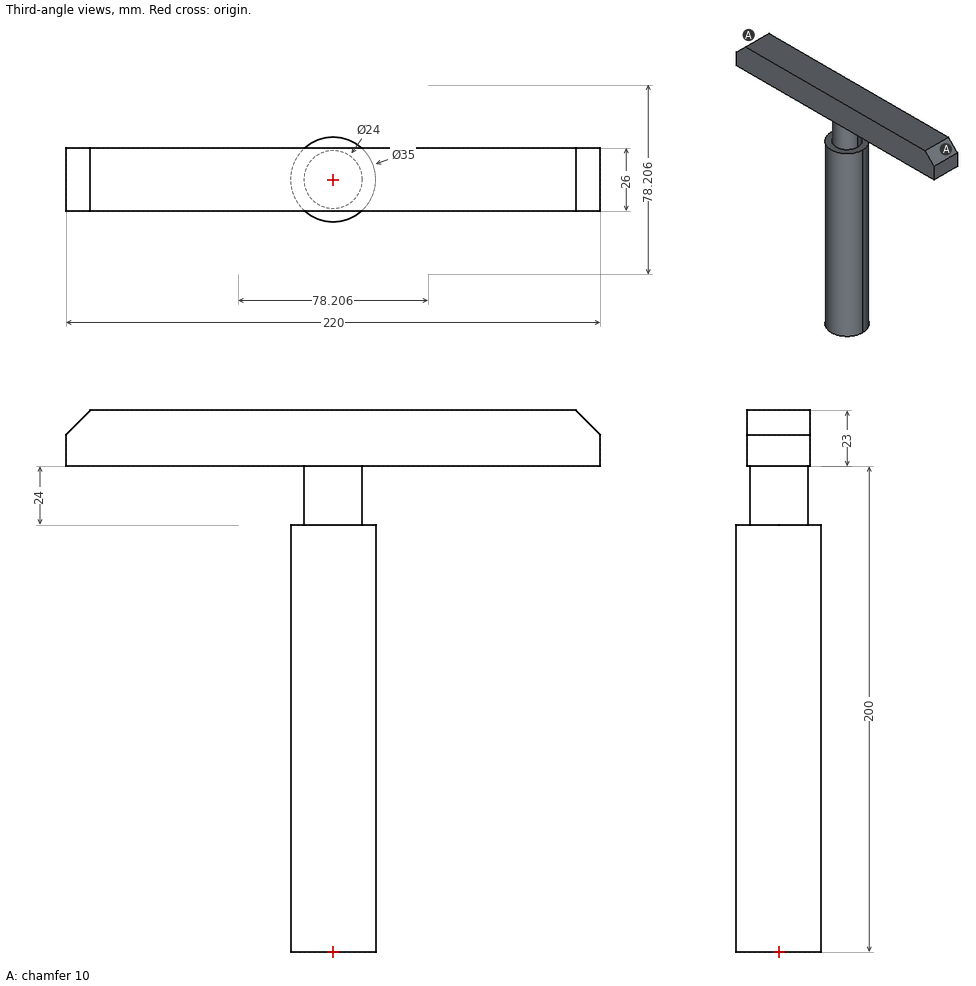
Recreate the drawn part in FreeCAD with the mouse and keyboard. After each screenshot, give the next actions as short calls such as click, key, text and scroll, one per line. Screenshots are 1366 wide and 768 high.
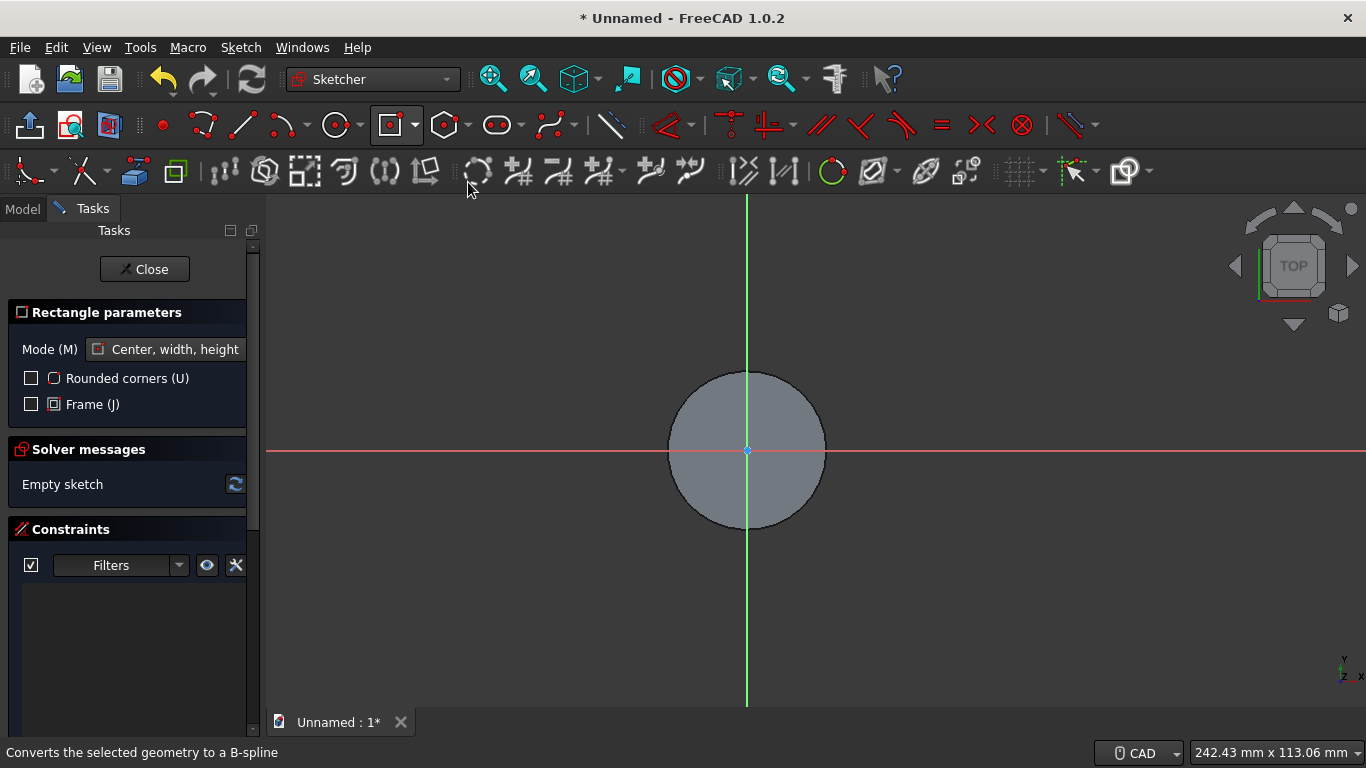
click(747, 450)
click(925, 273)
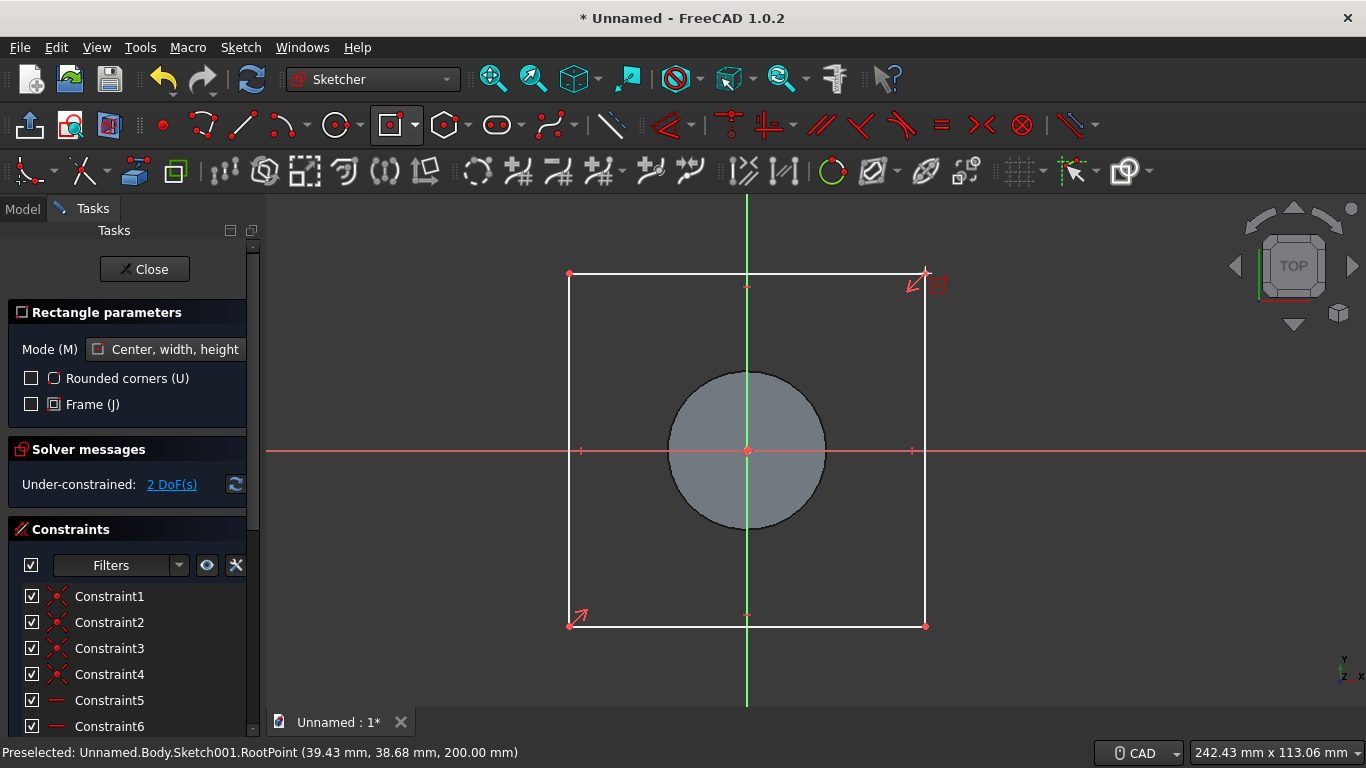
click(336, 126)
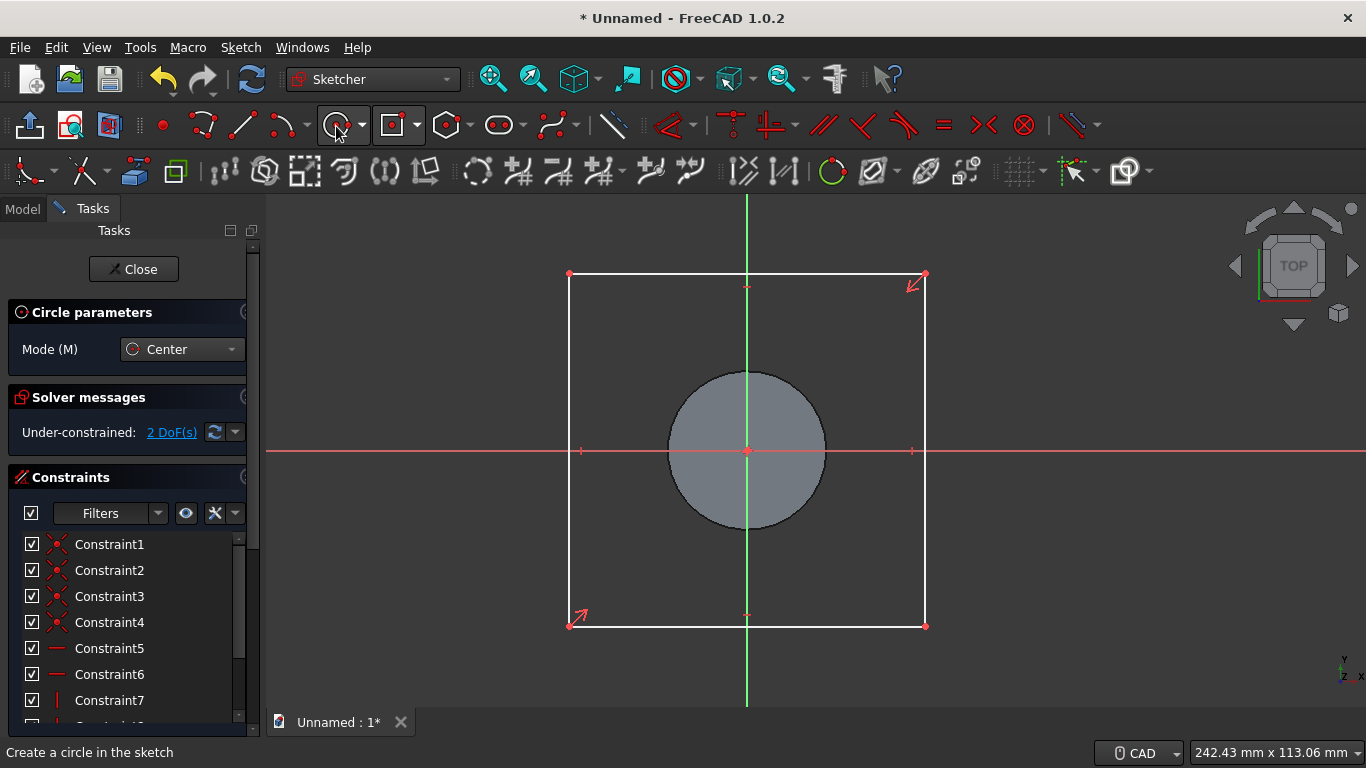
click(747, 450)
click(786, 412)
key(Escape)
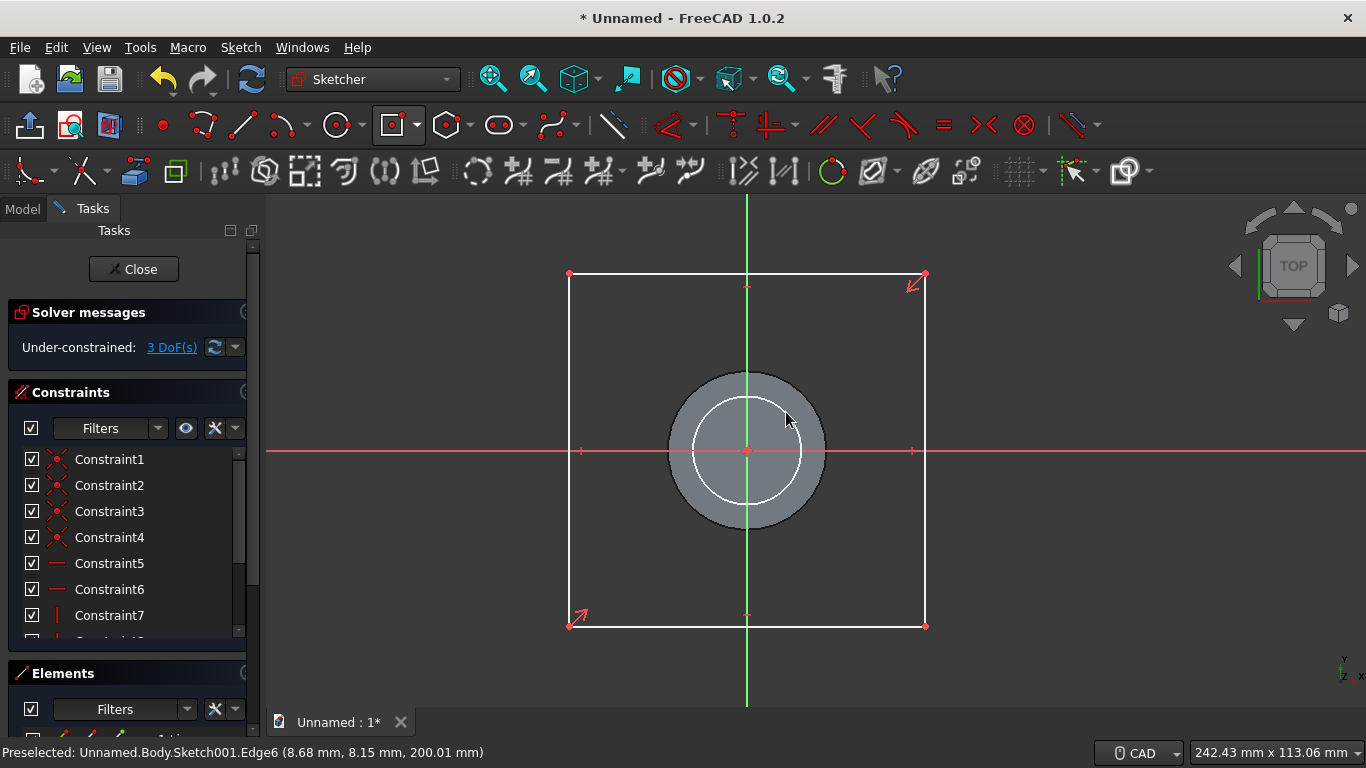
click(668, 126)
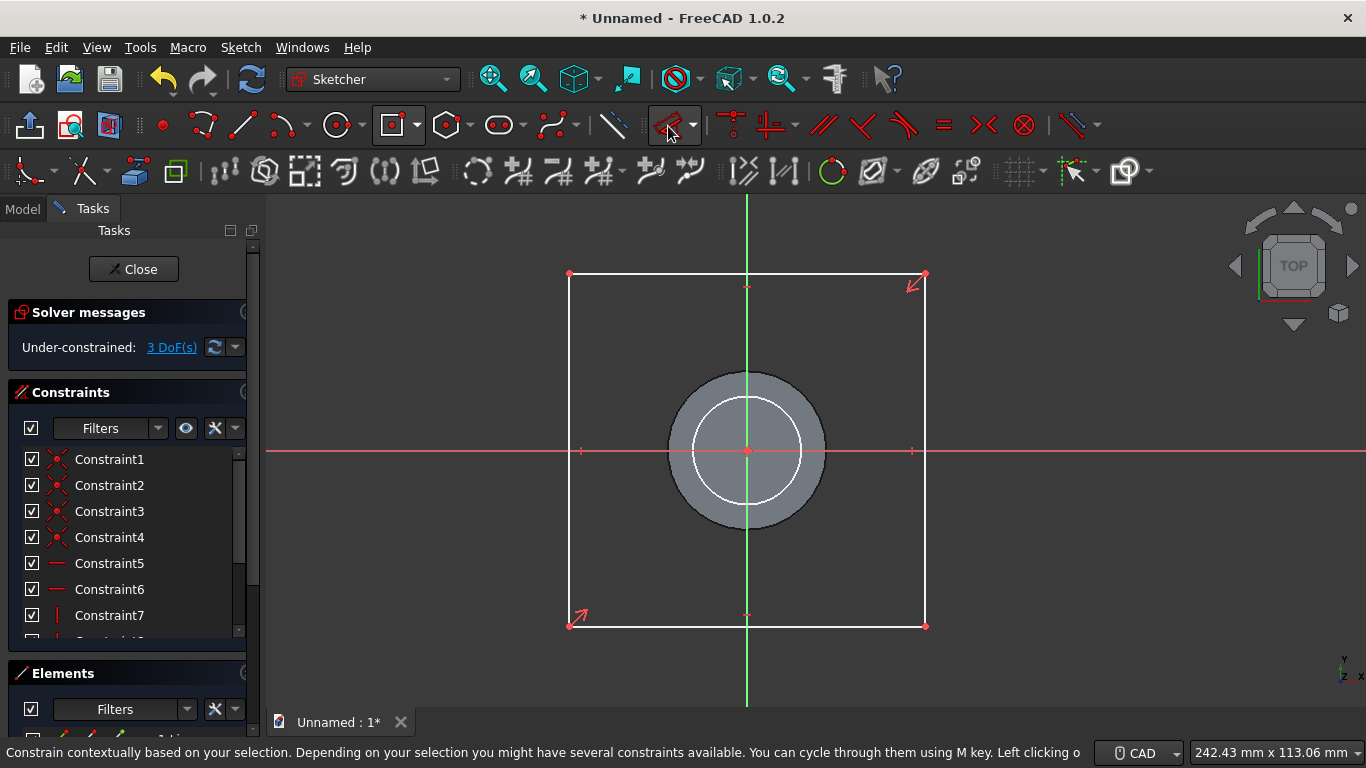
click(785, 412)
click(807, 389)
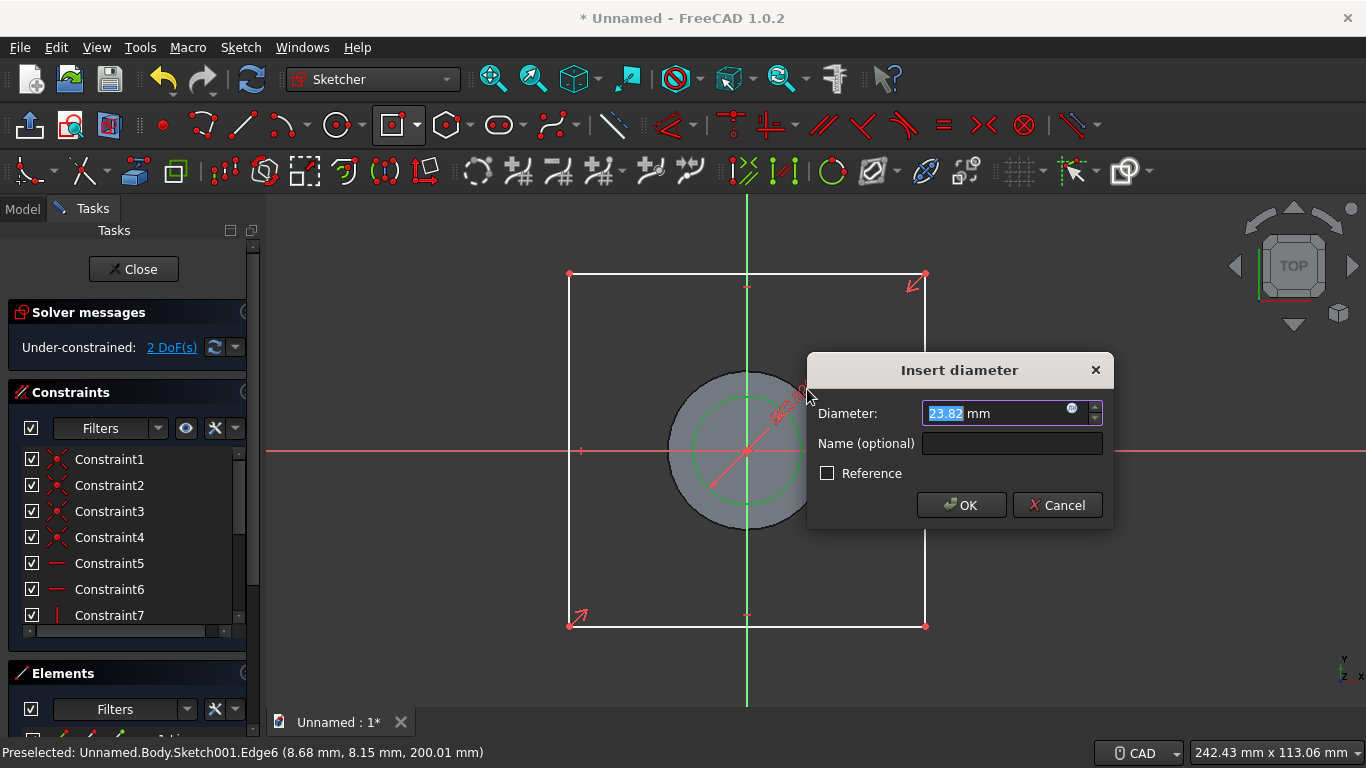
text(24)
key(Return)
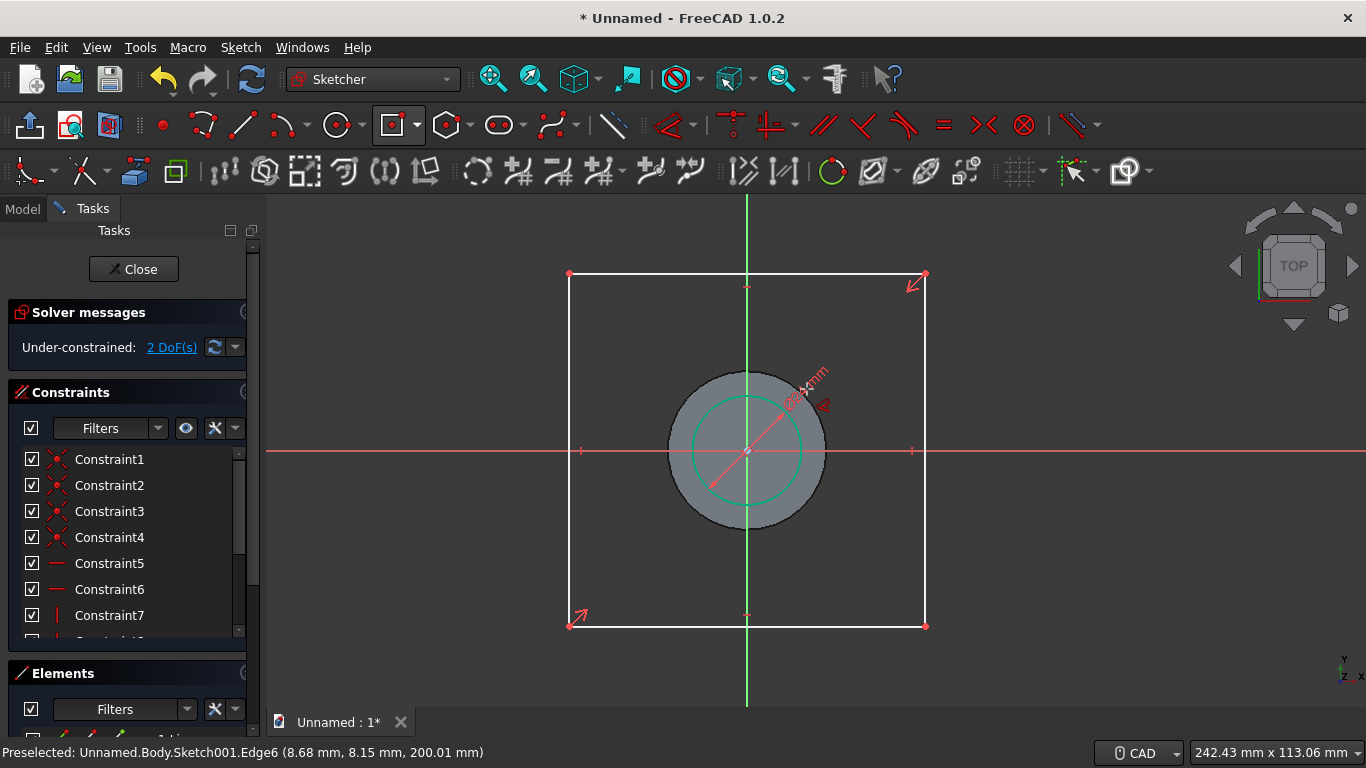
click(676, 627)
click(665, 661)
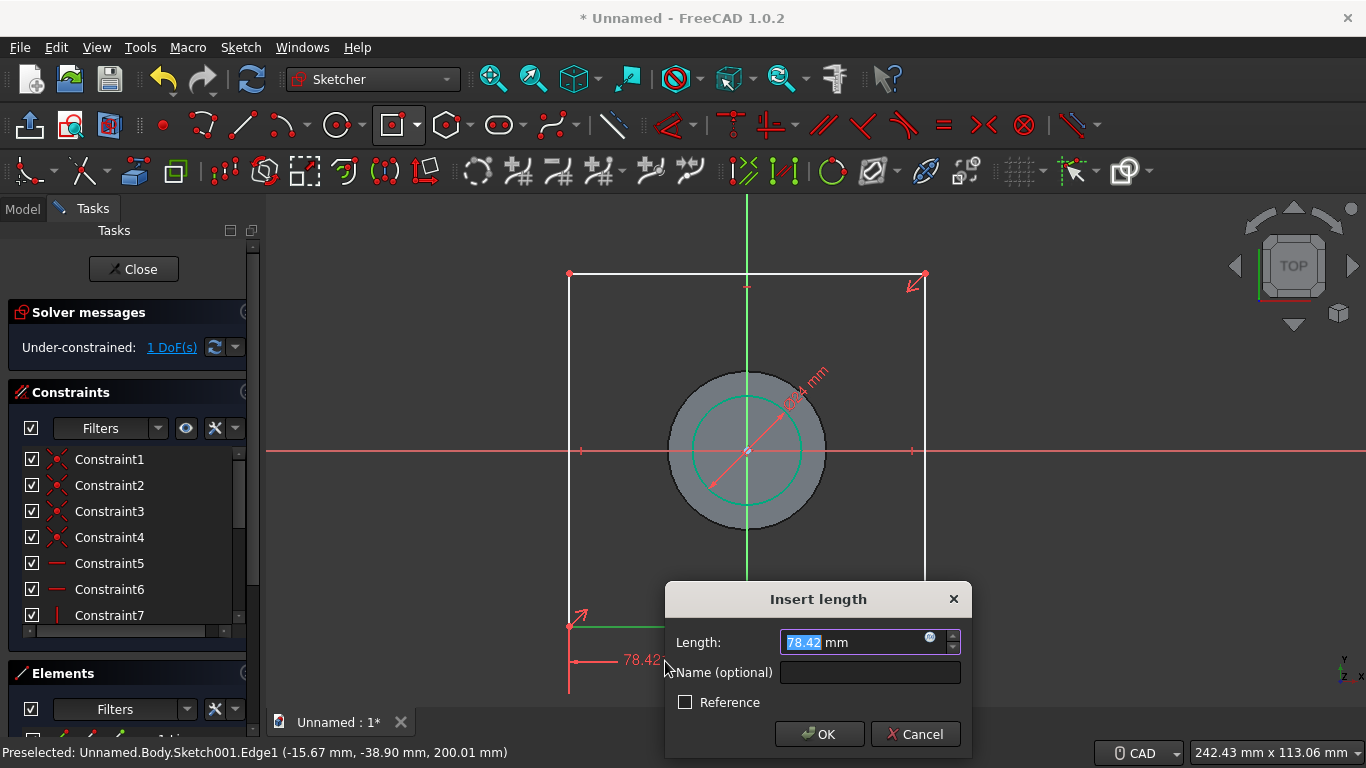
text(78.206)
key(Return)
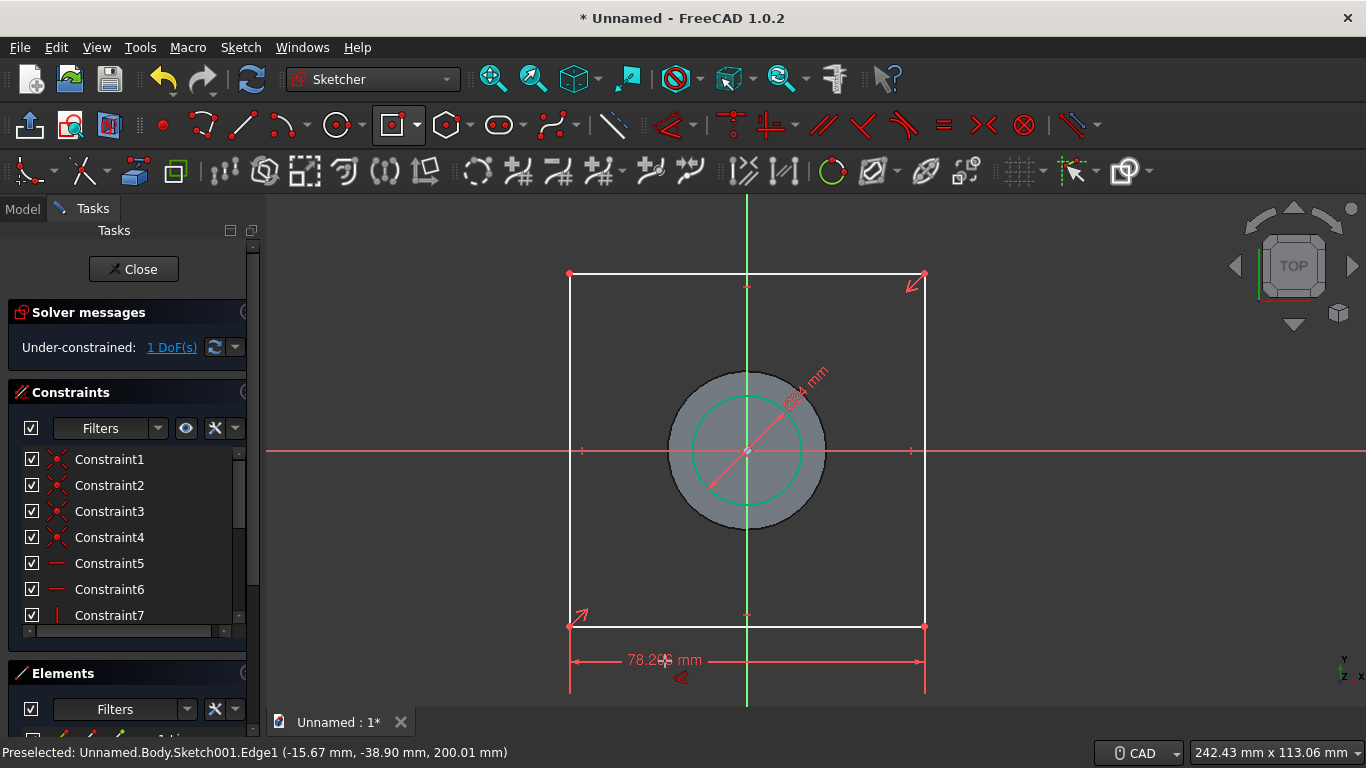
click(925, 521)
click(959, 369)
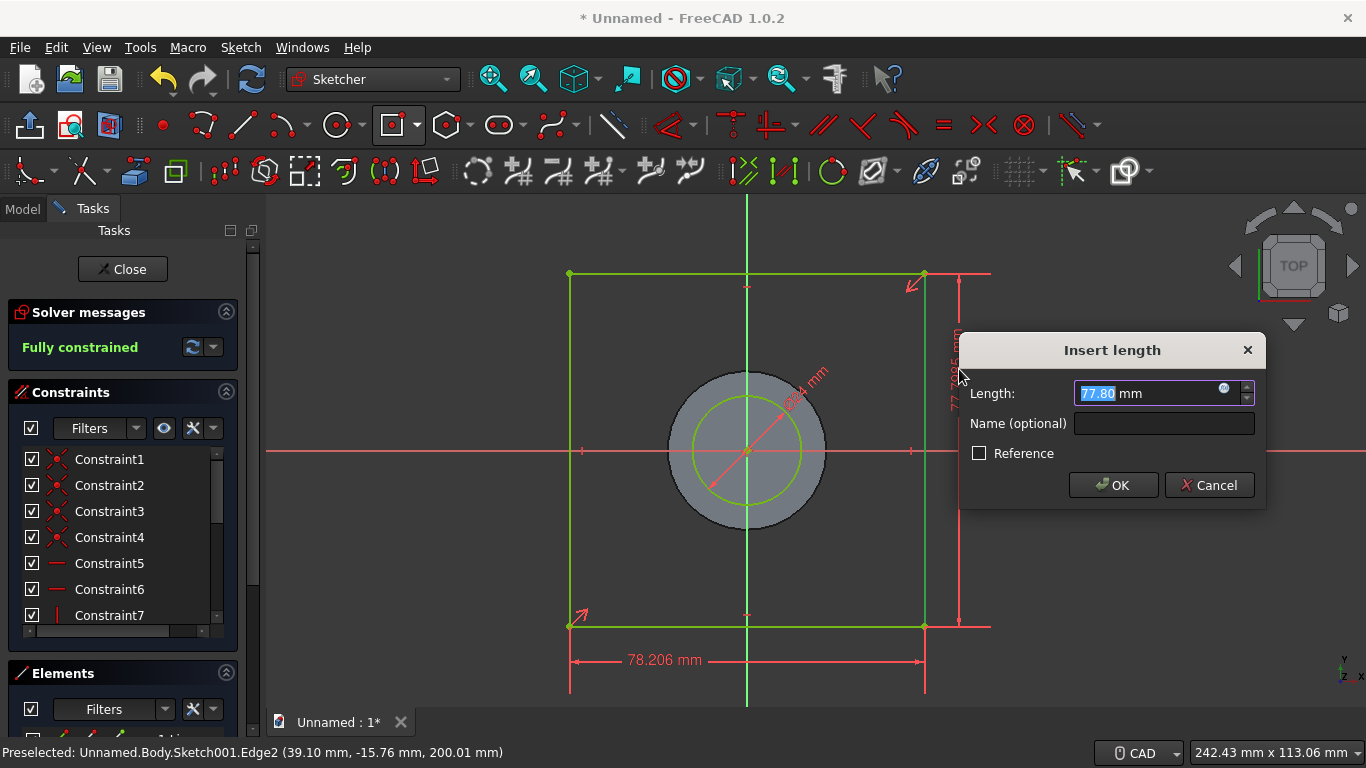
text(78.206)
key(Return)
key(Escape)